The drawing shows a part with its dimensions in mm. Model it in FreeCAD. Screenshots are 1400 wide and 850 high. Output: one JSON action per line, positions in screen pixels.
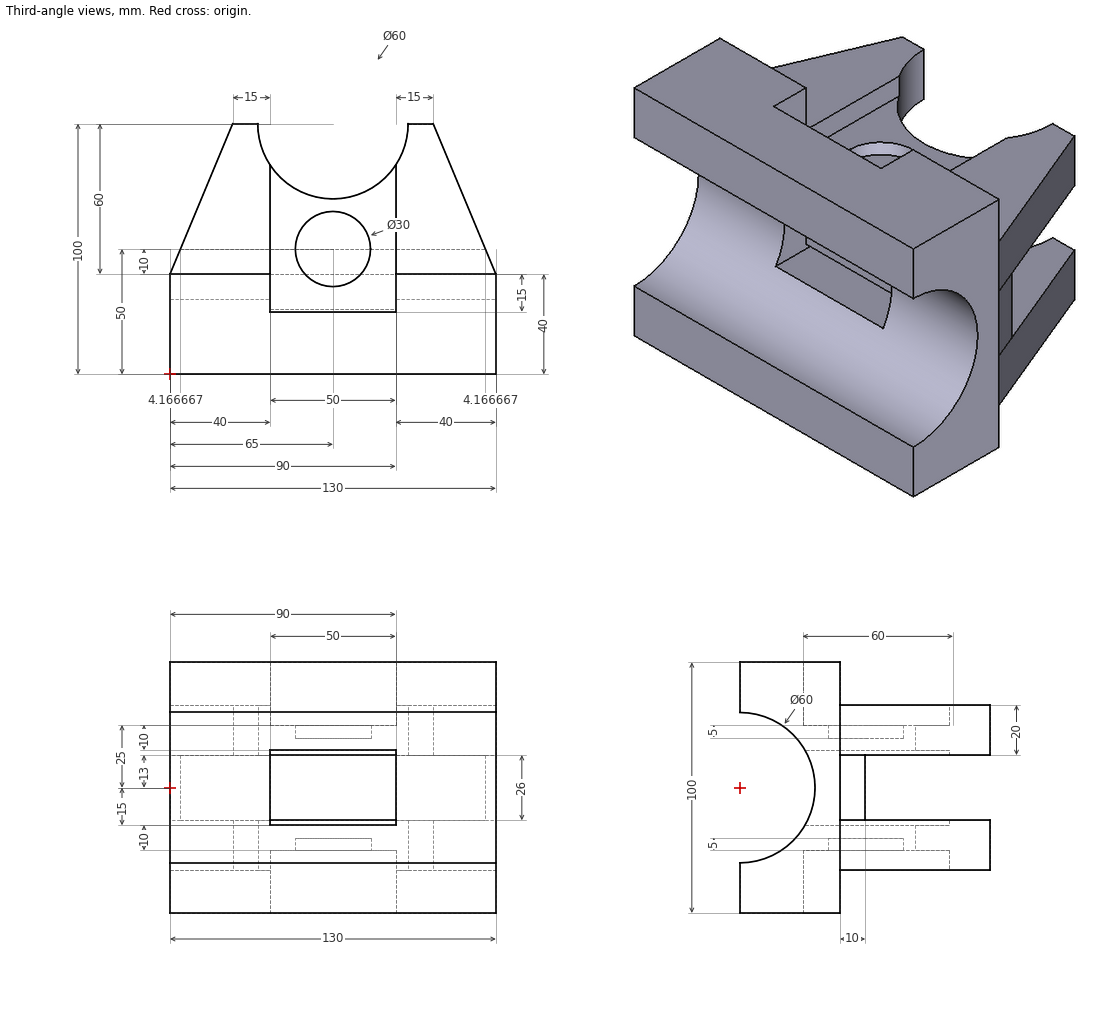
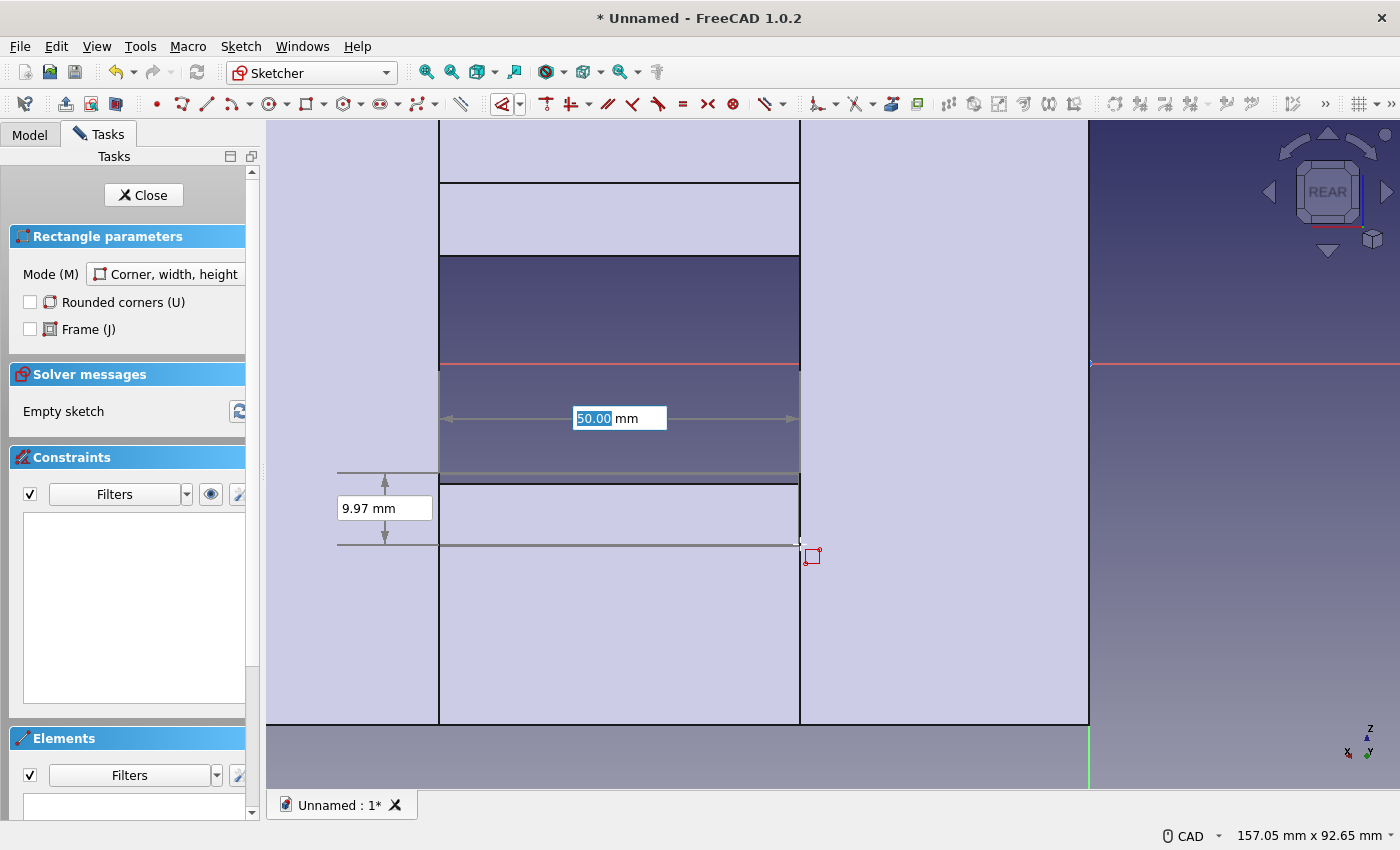
{"action": "type", "text": "50"}
{"action": "key", "text": "Tab"}
{"action": "type", "text": "10"}
{"action": "key", "text": "Return"}
{"action": "key", "text": "Escape"}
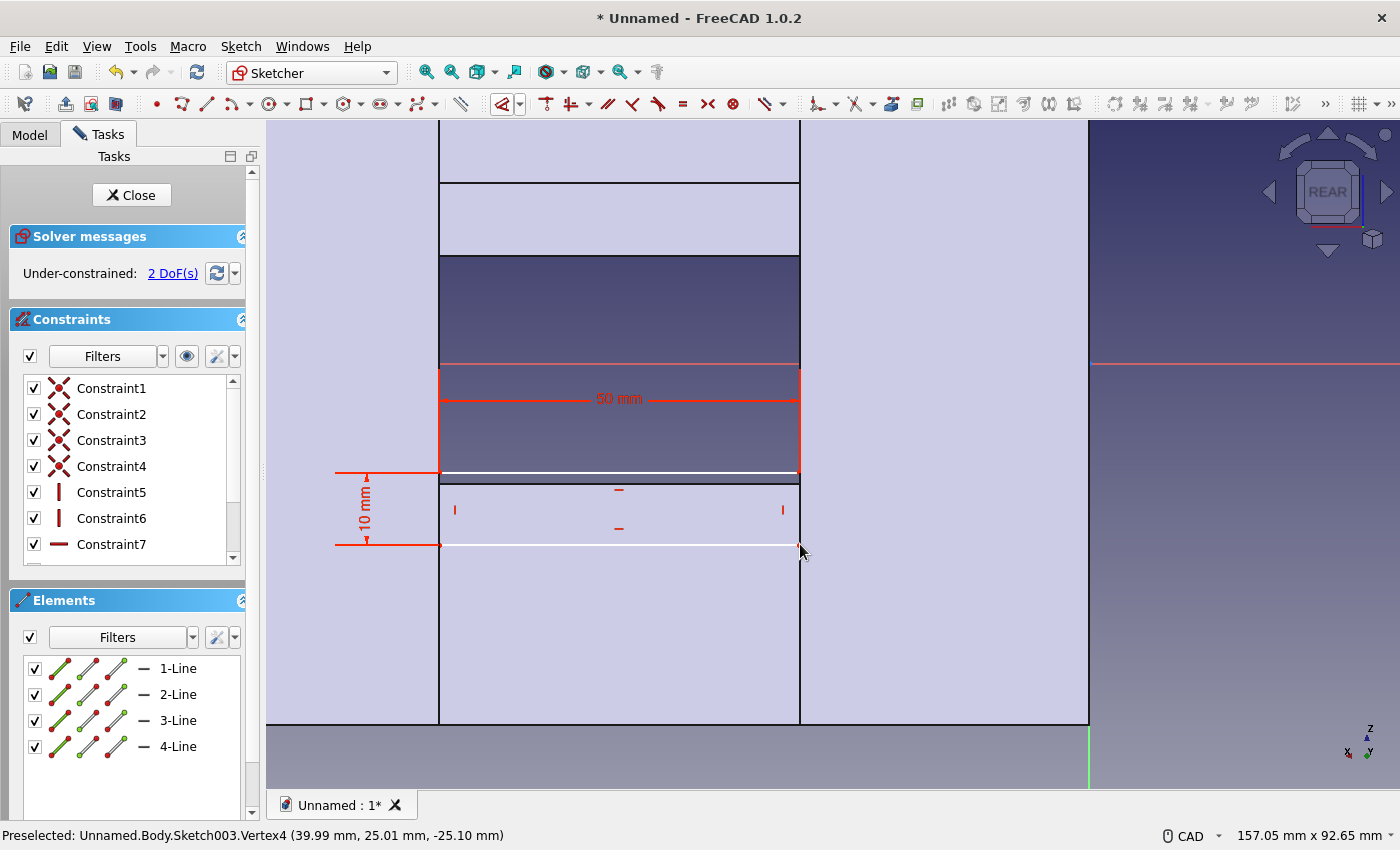
{"action": "left_click", "coordinate": [439, 473]}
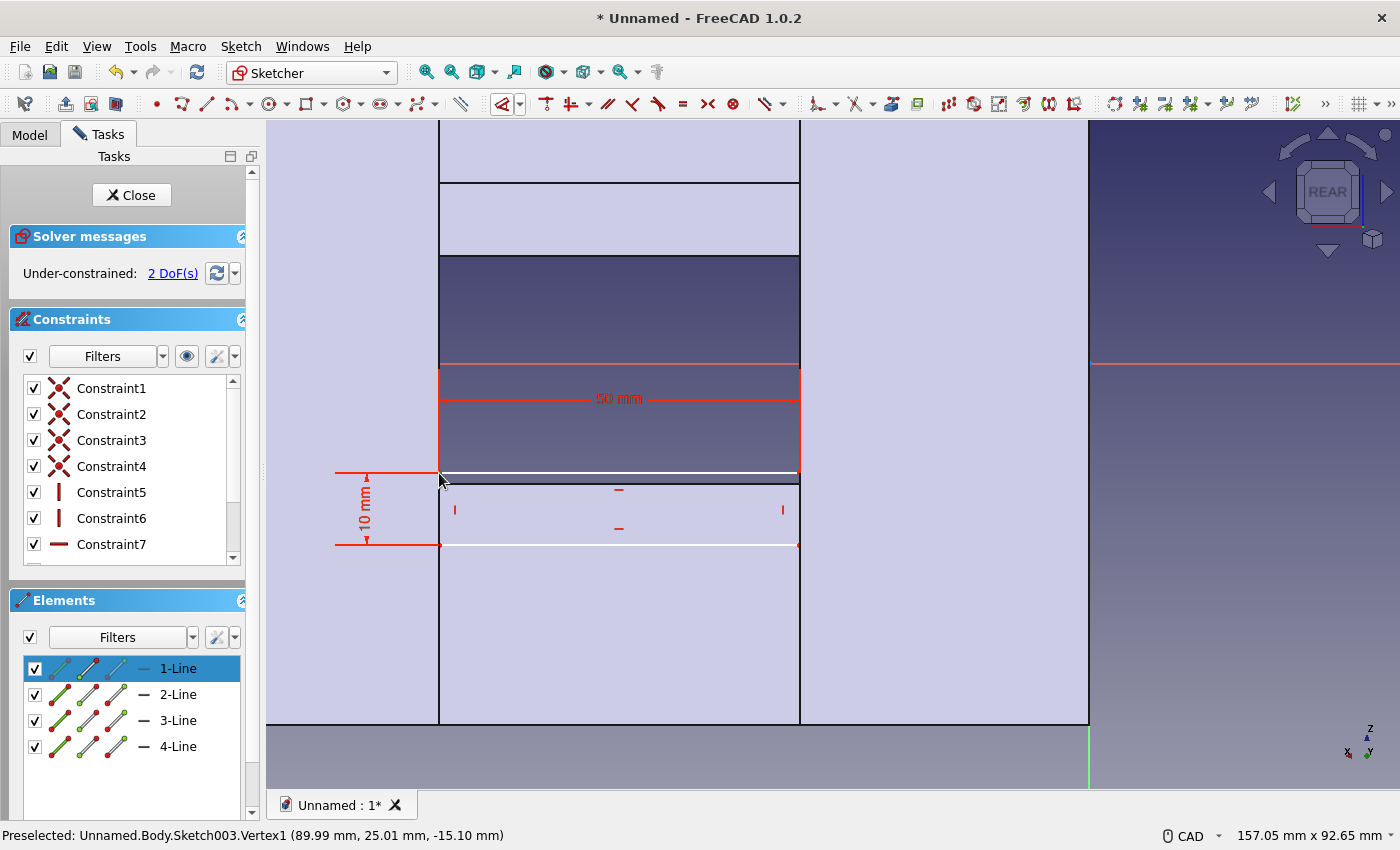
{"action": "left_click", "coordinate": [520, 104]}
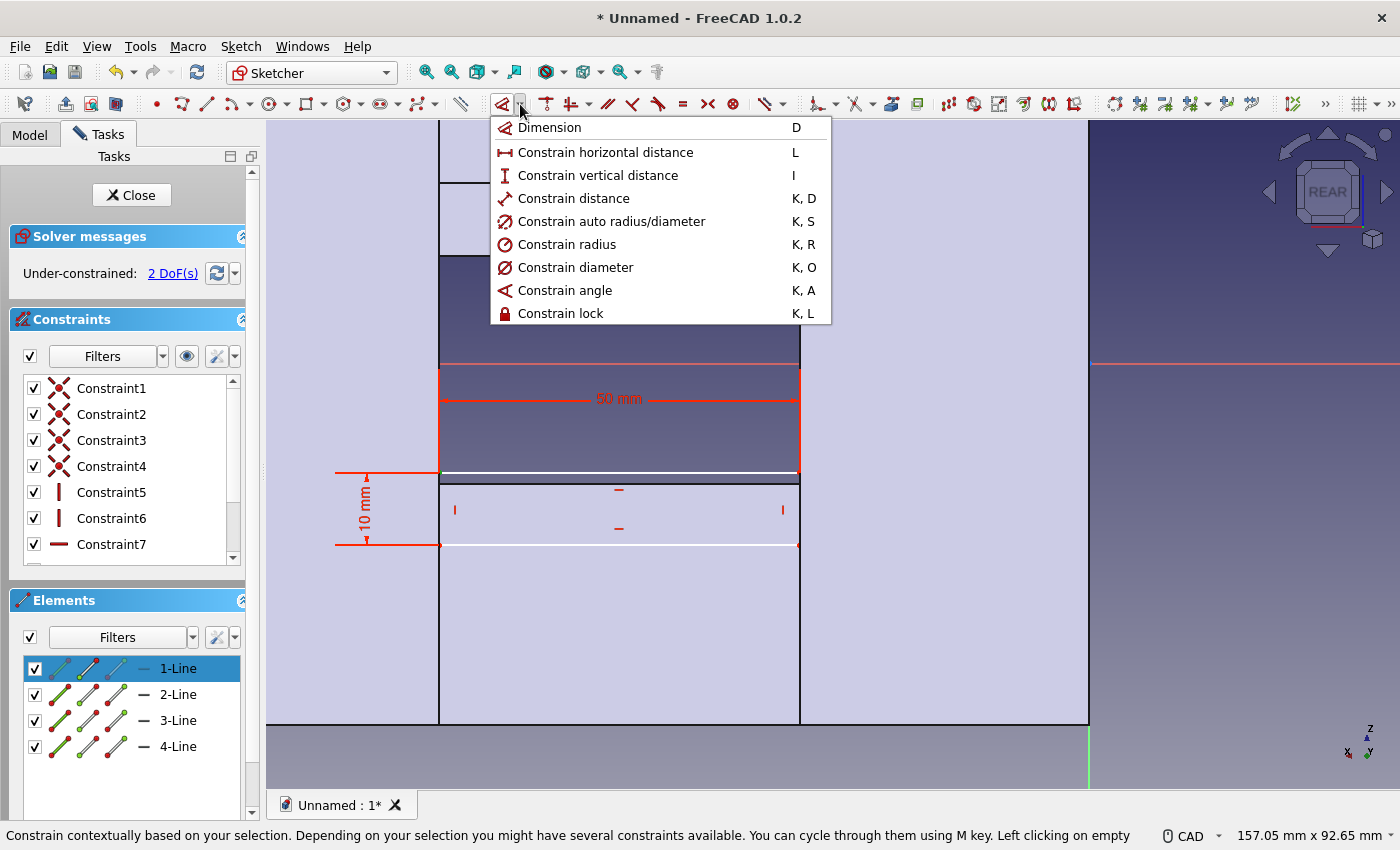
{"action": "left_click", "coordinate": [661, 152]}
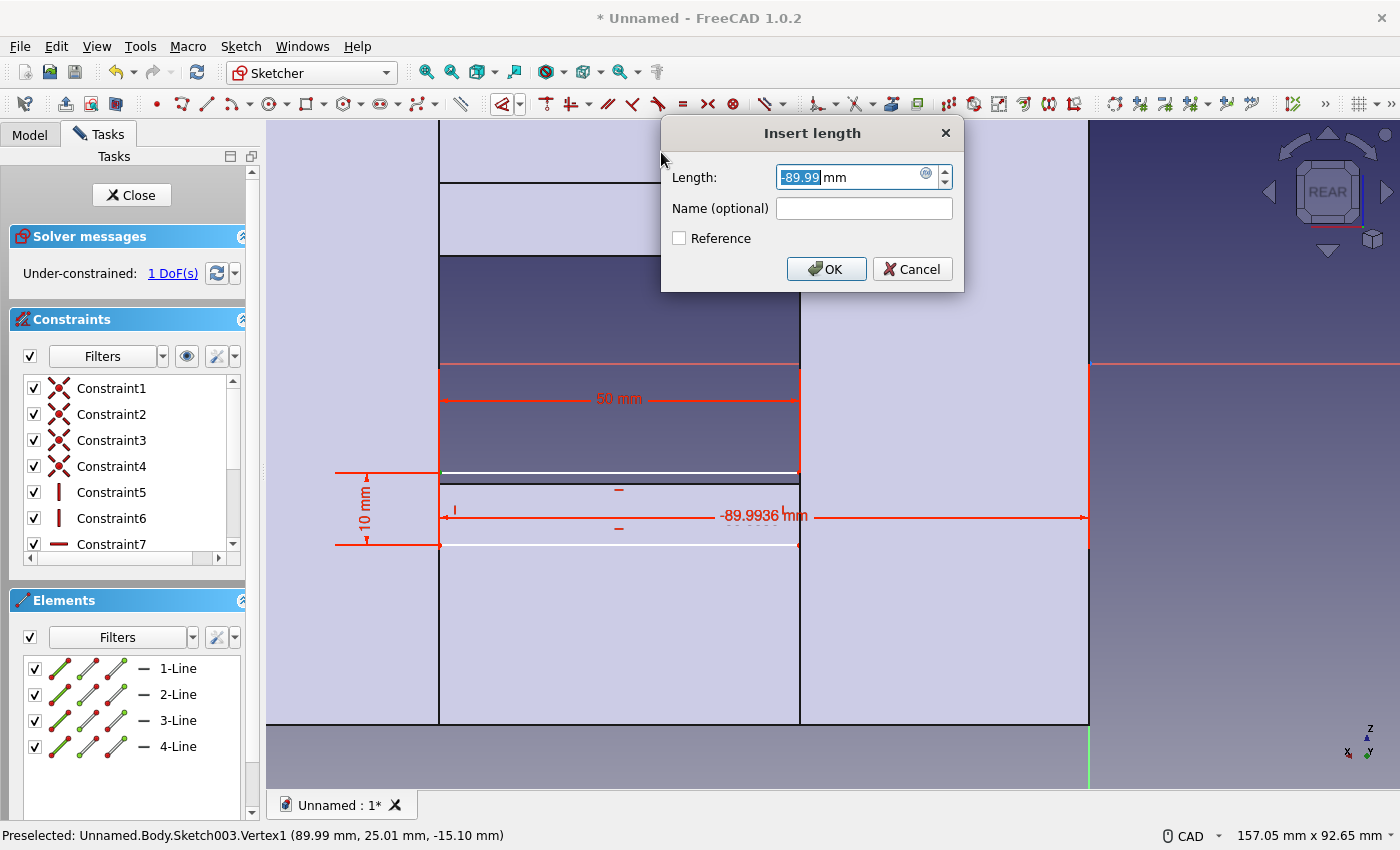
{"action": "type", "text": "-90"}
{"action": "key", "text": "Return"}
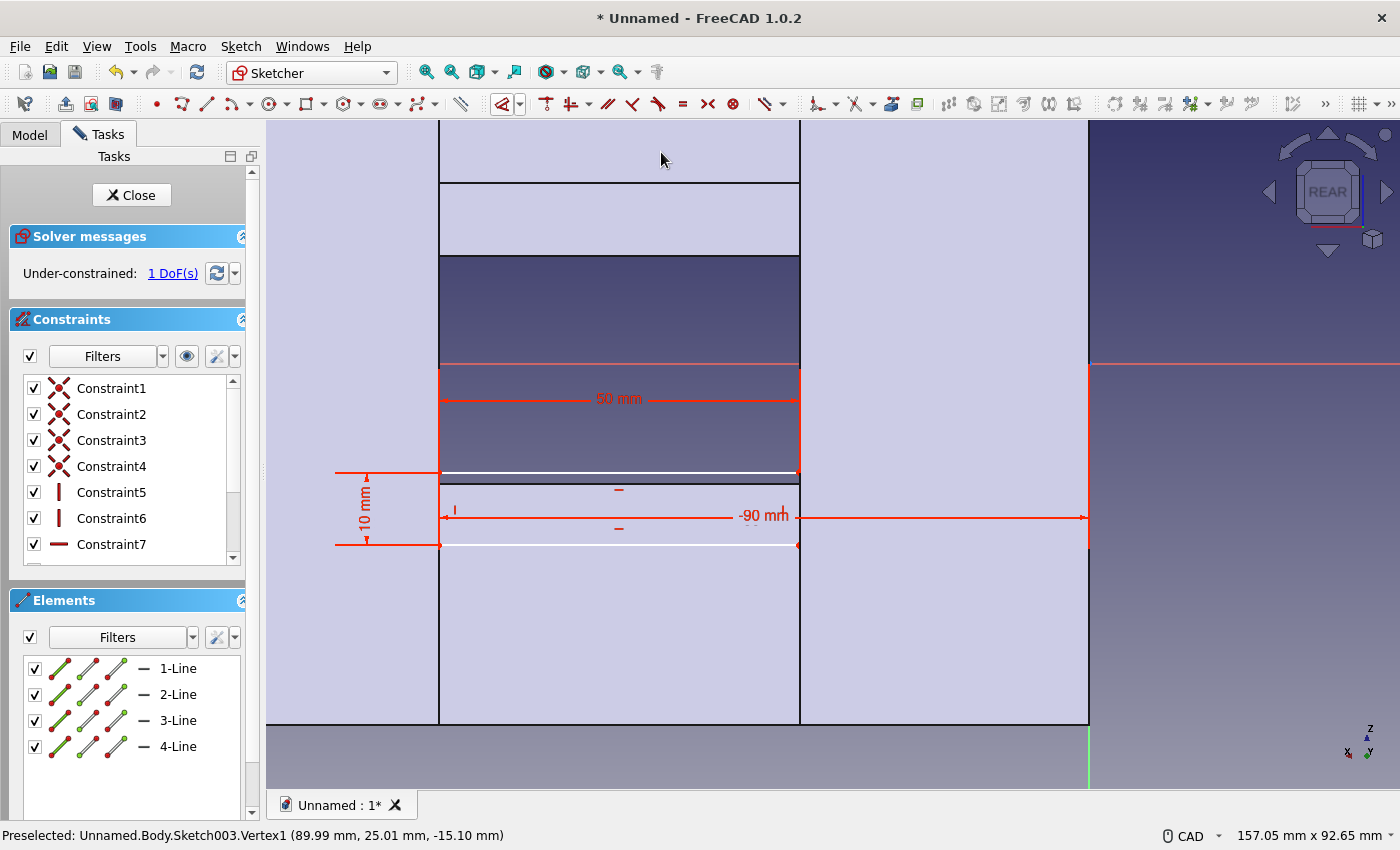
{"action": "left_click", "coordinate": [439, 473]}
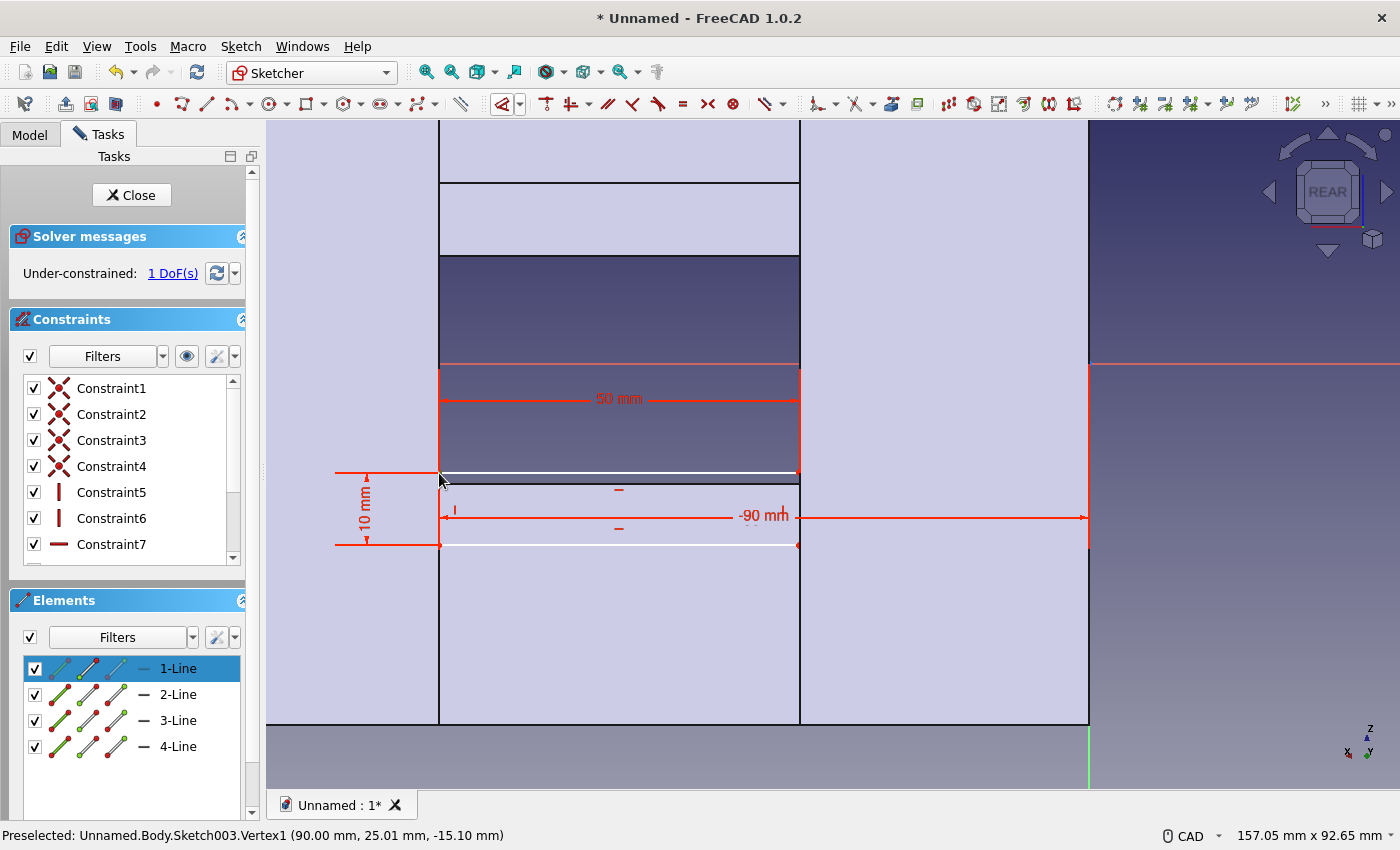
{"action": "left_click", "coordinate": [520, 104]}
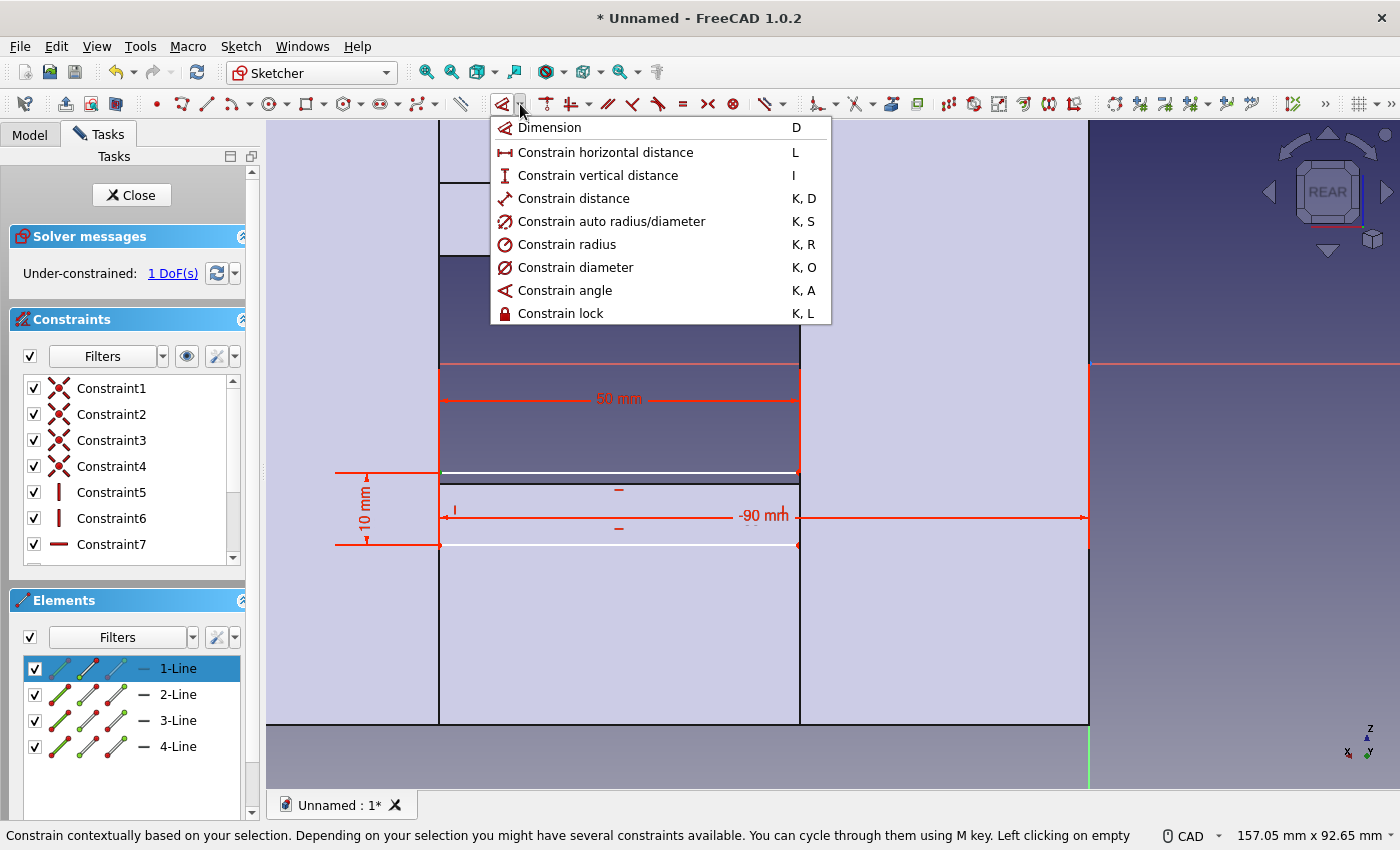
{"action": "left_click", "coordinate": [661, 176]}